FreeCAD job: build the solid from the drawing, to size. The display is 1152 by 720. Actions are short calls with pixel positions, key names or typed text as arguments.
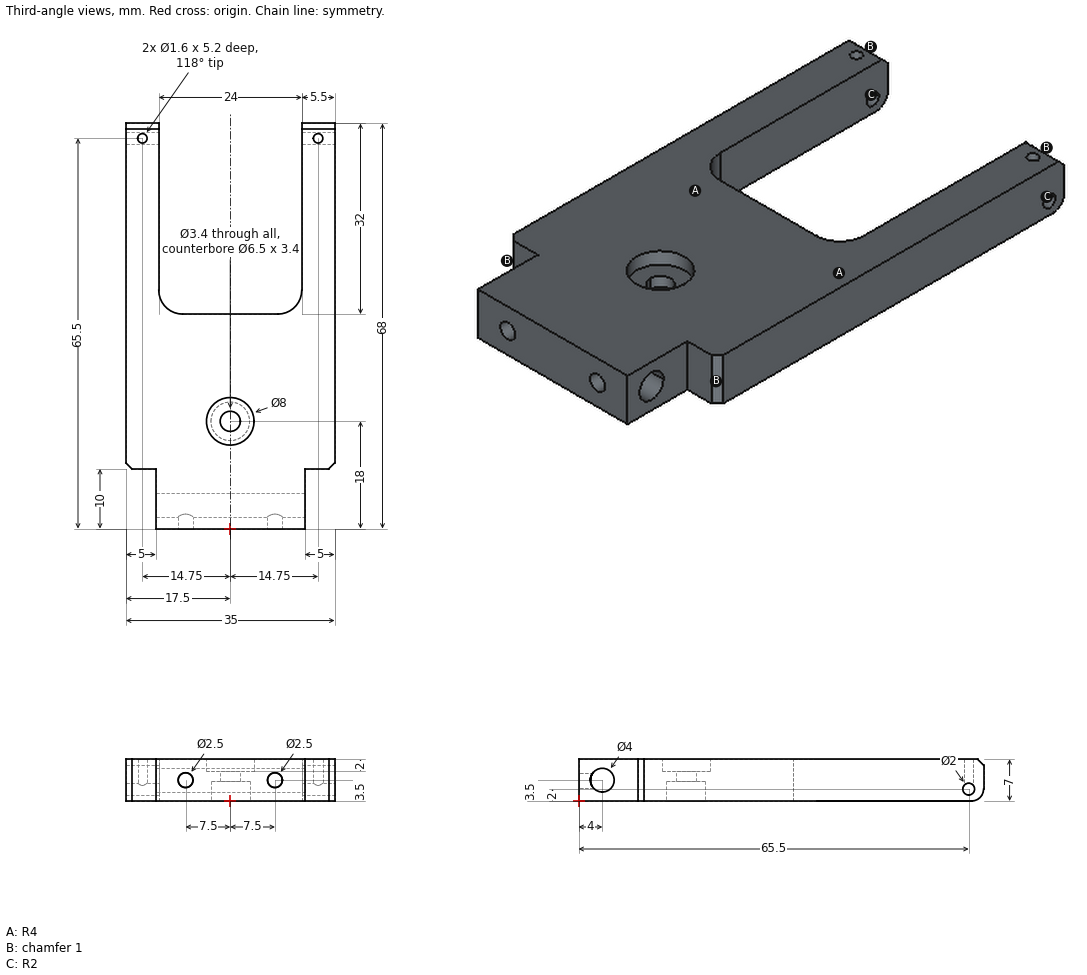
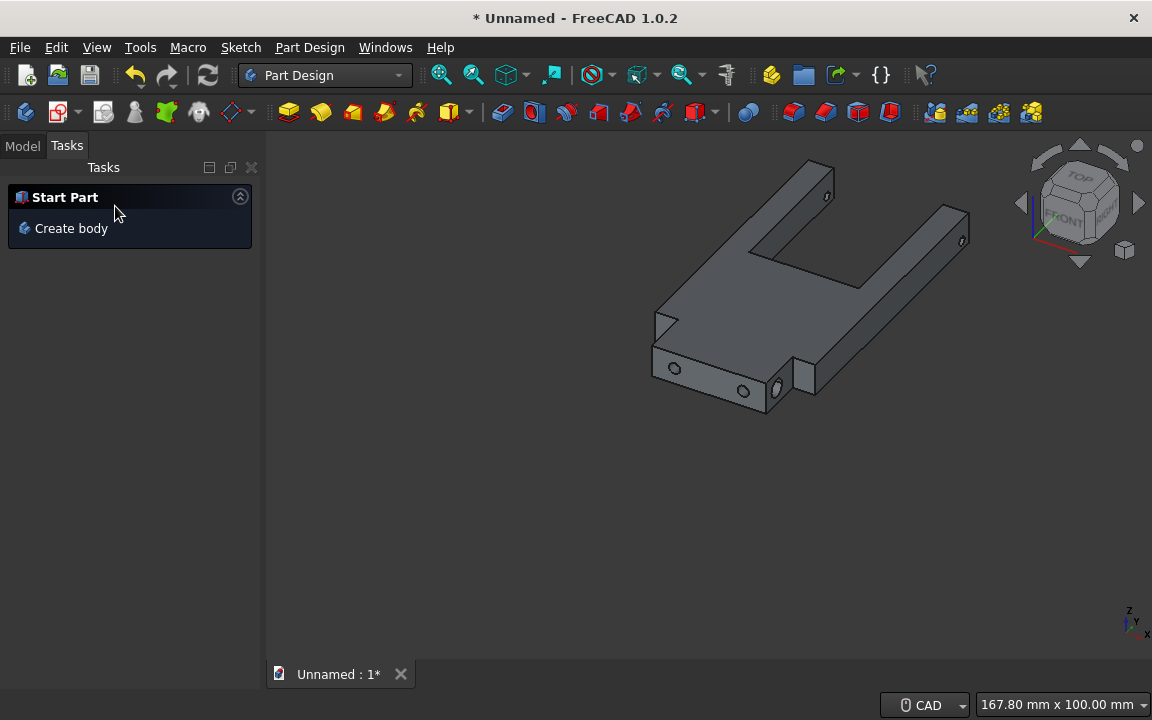
key(0)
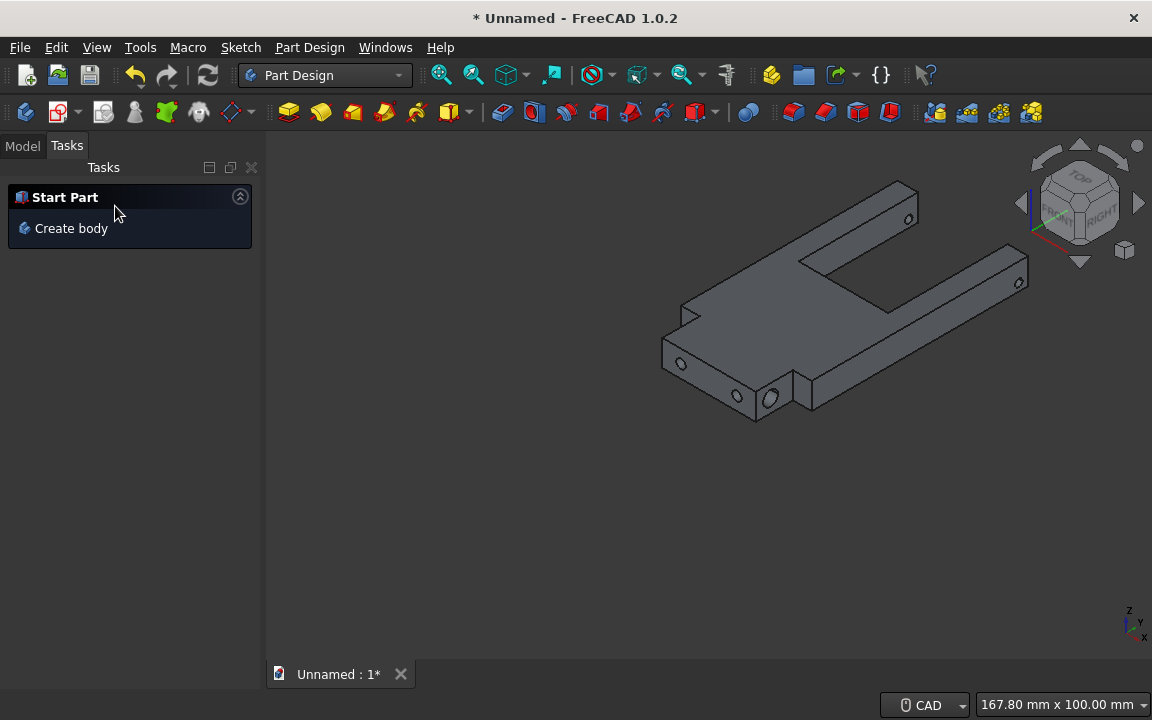
key(2)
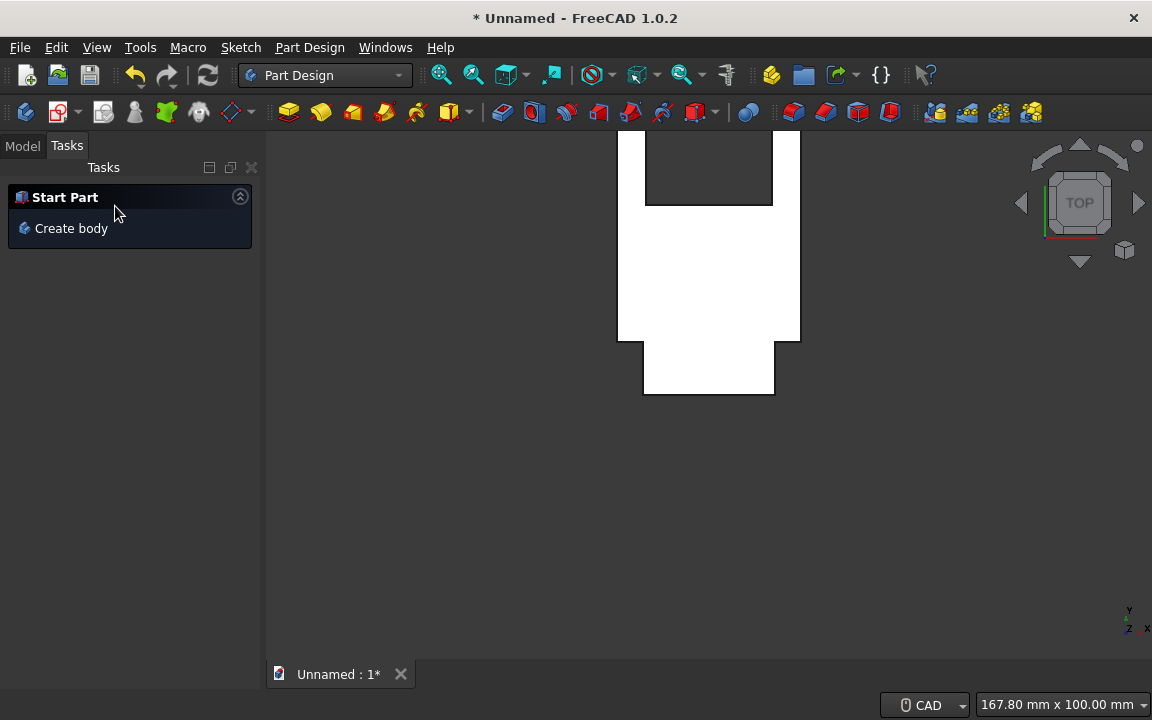
key(v)
key(f)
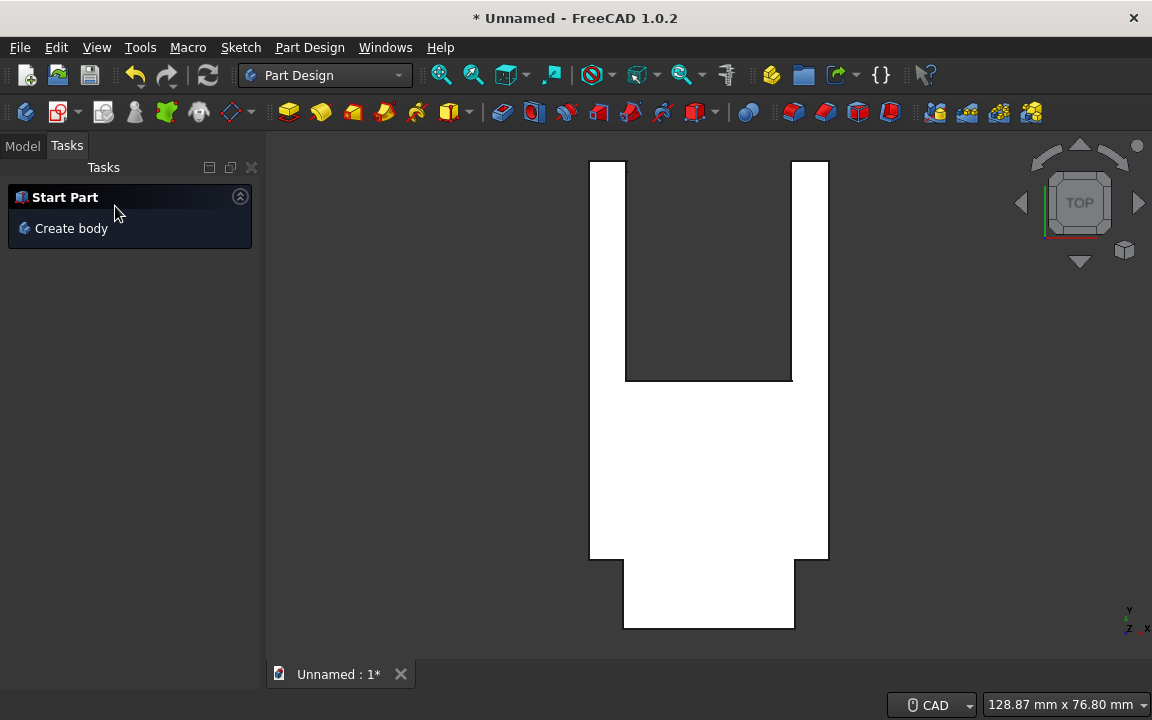
key(1)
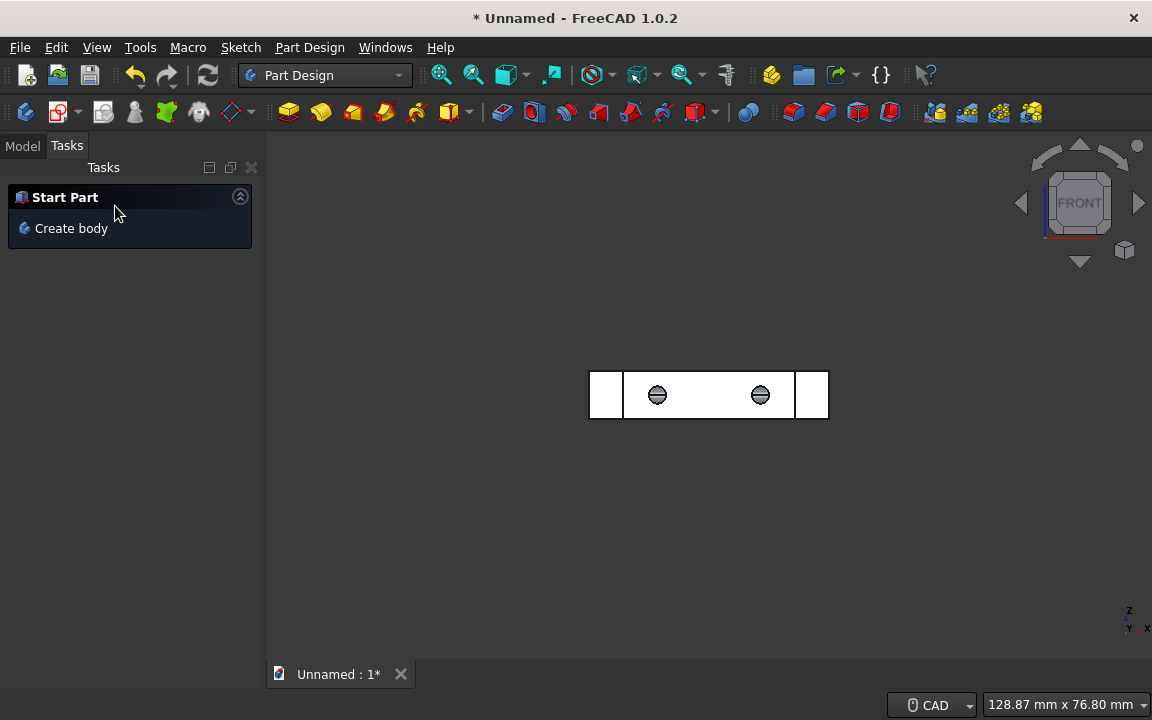
key(v)
key(f)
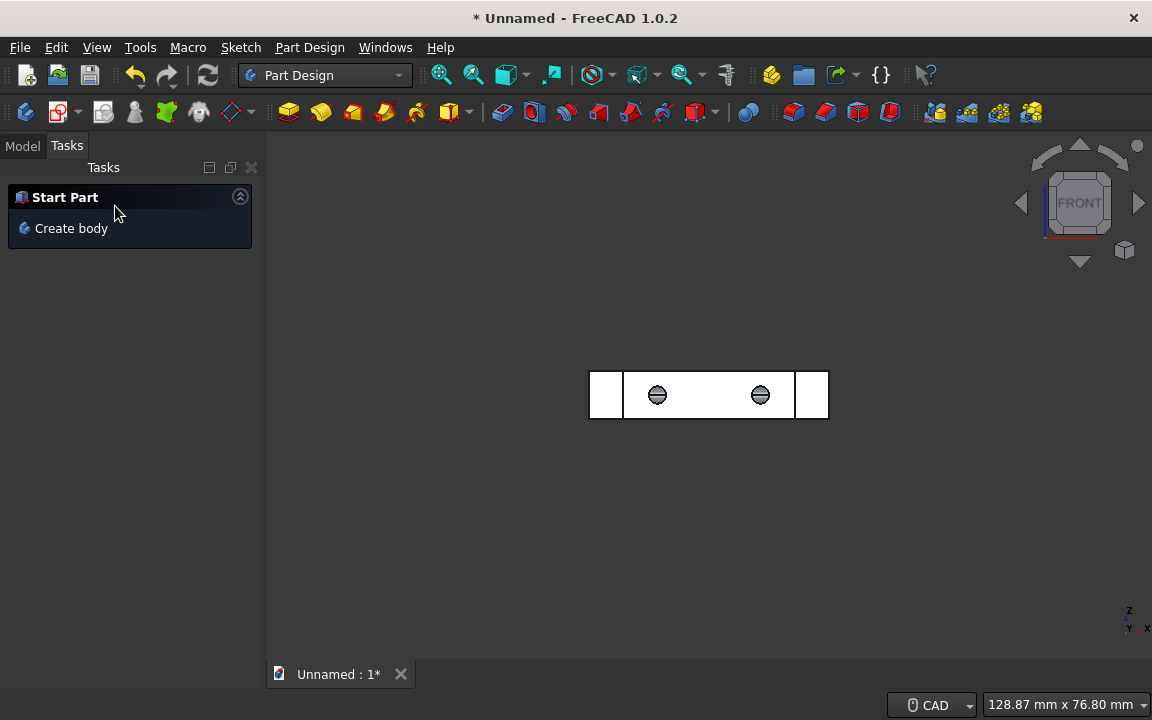
key(3)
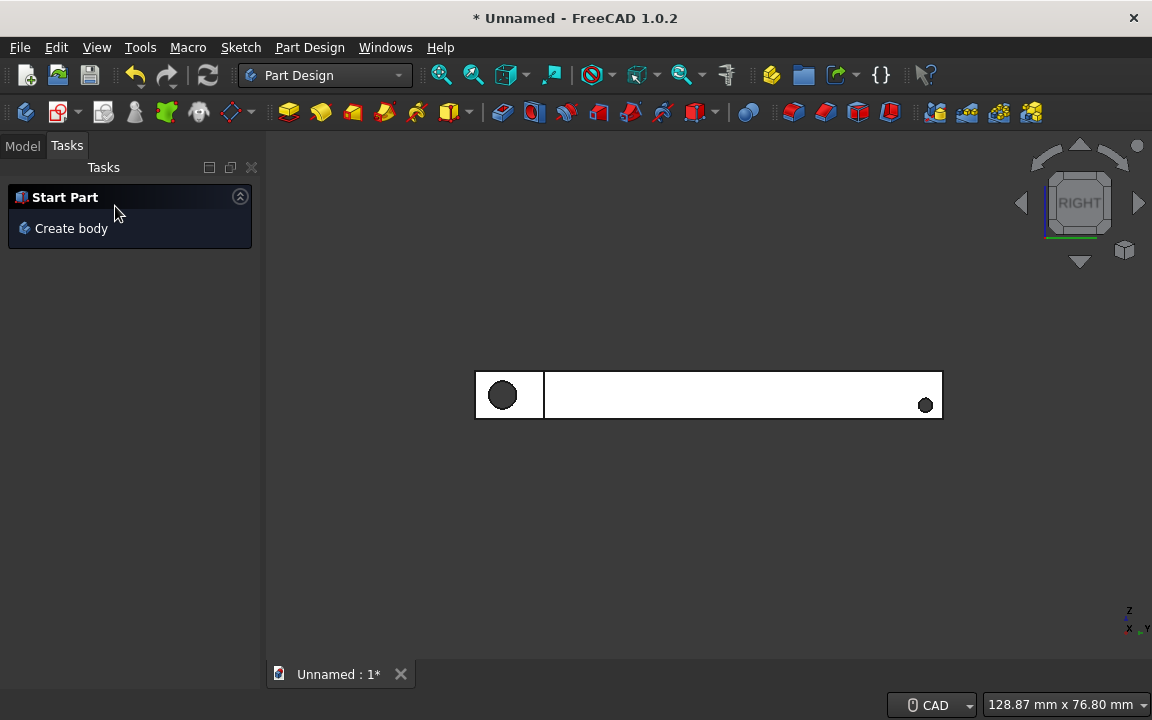
key(5)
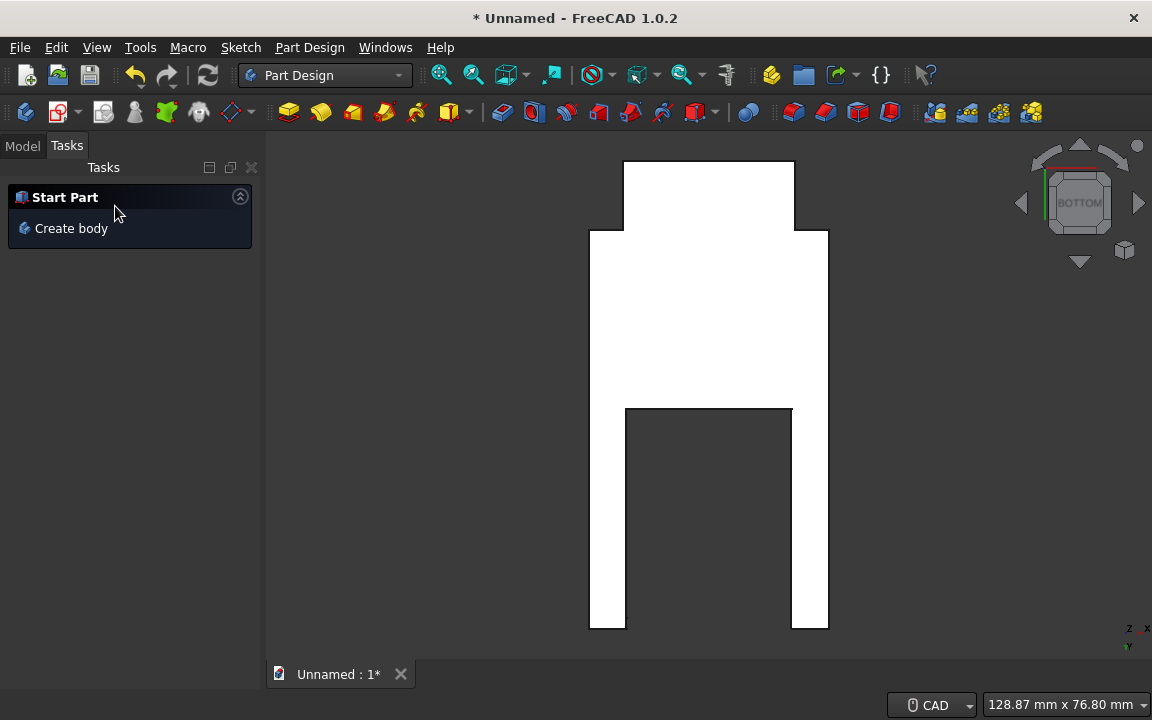
key(4)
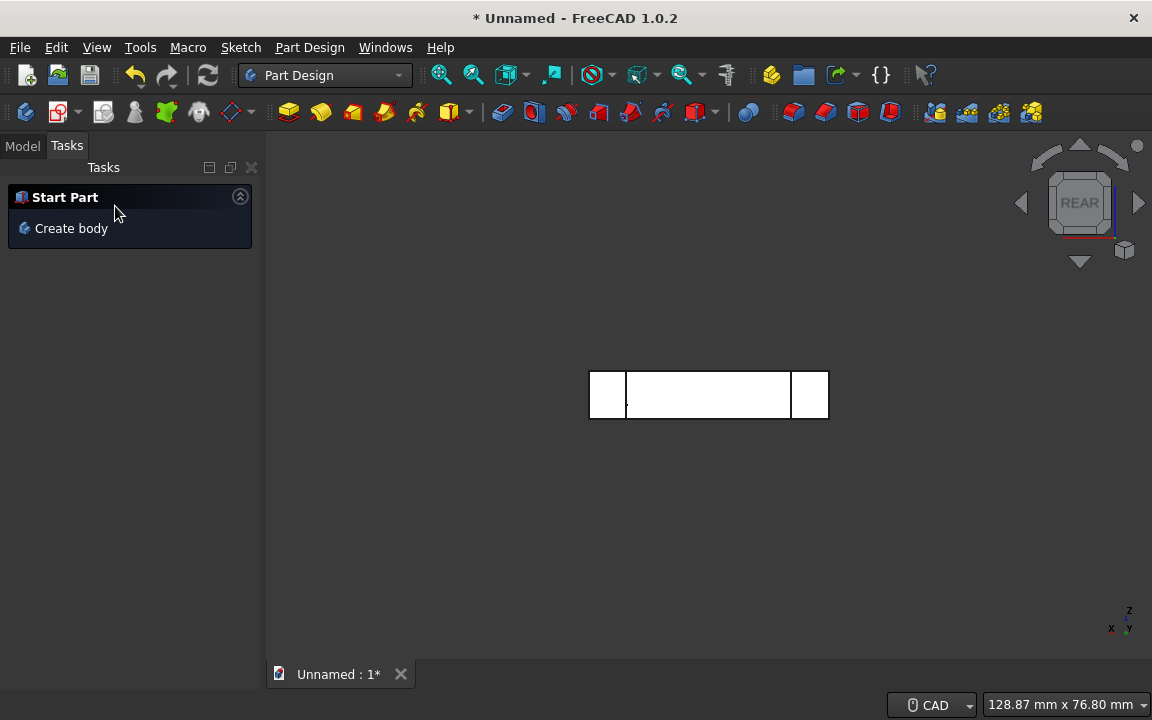
click(442, 76)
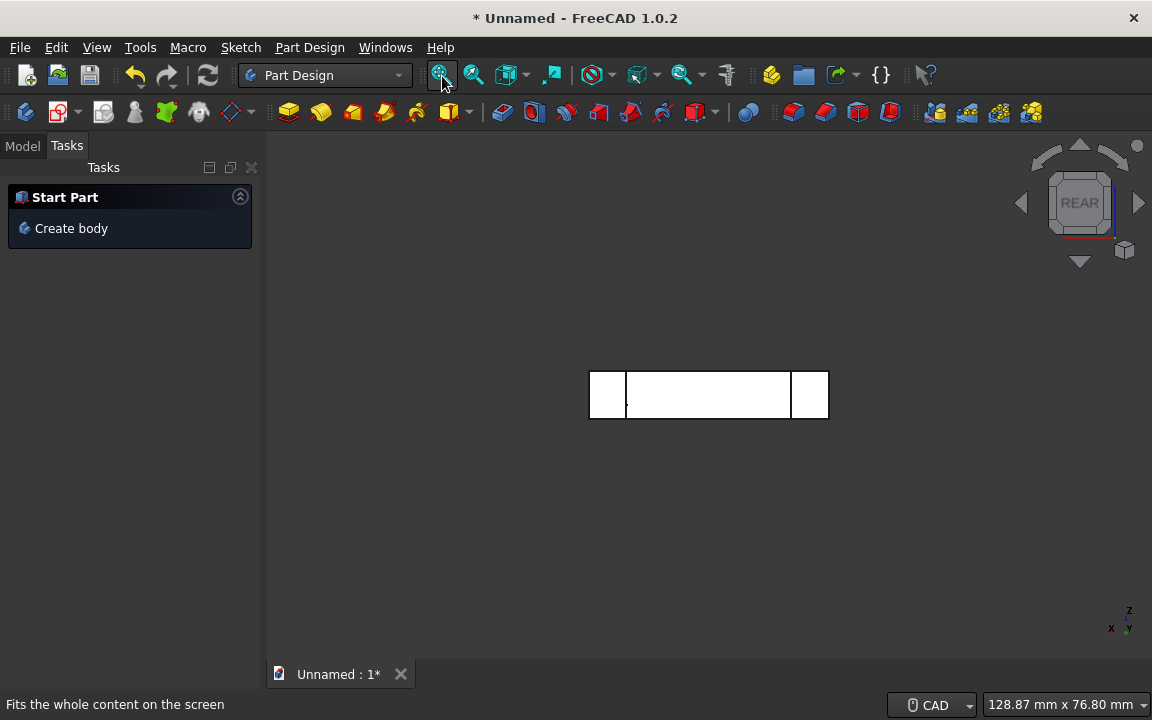
key(6)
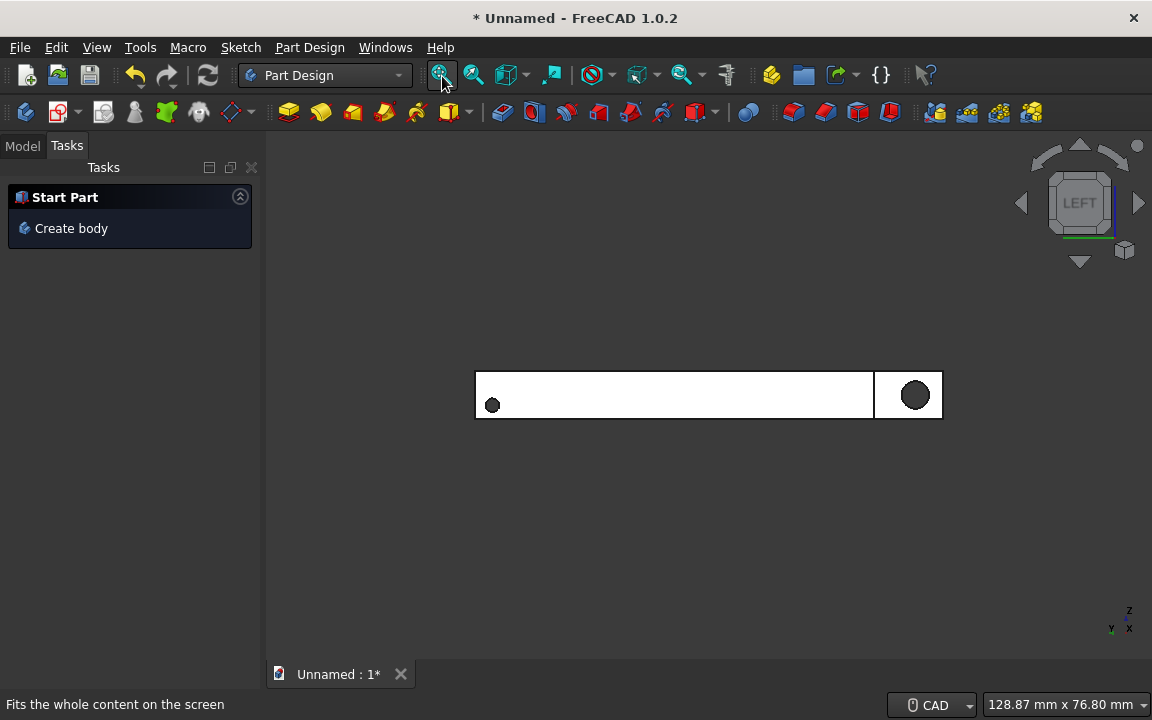
key(v)
key(3)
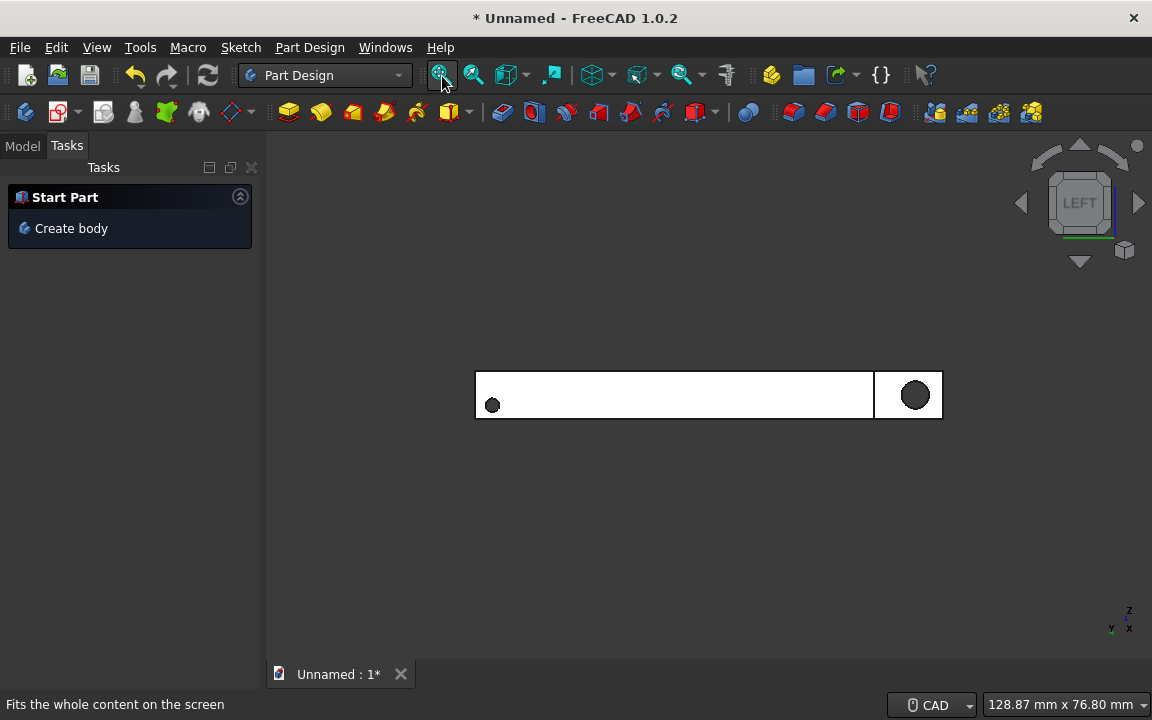
key(0)